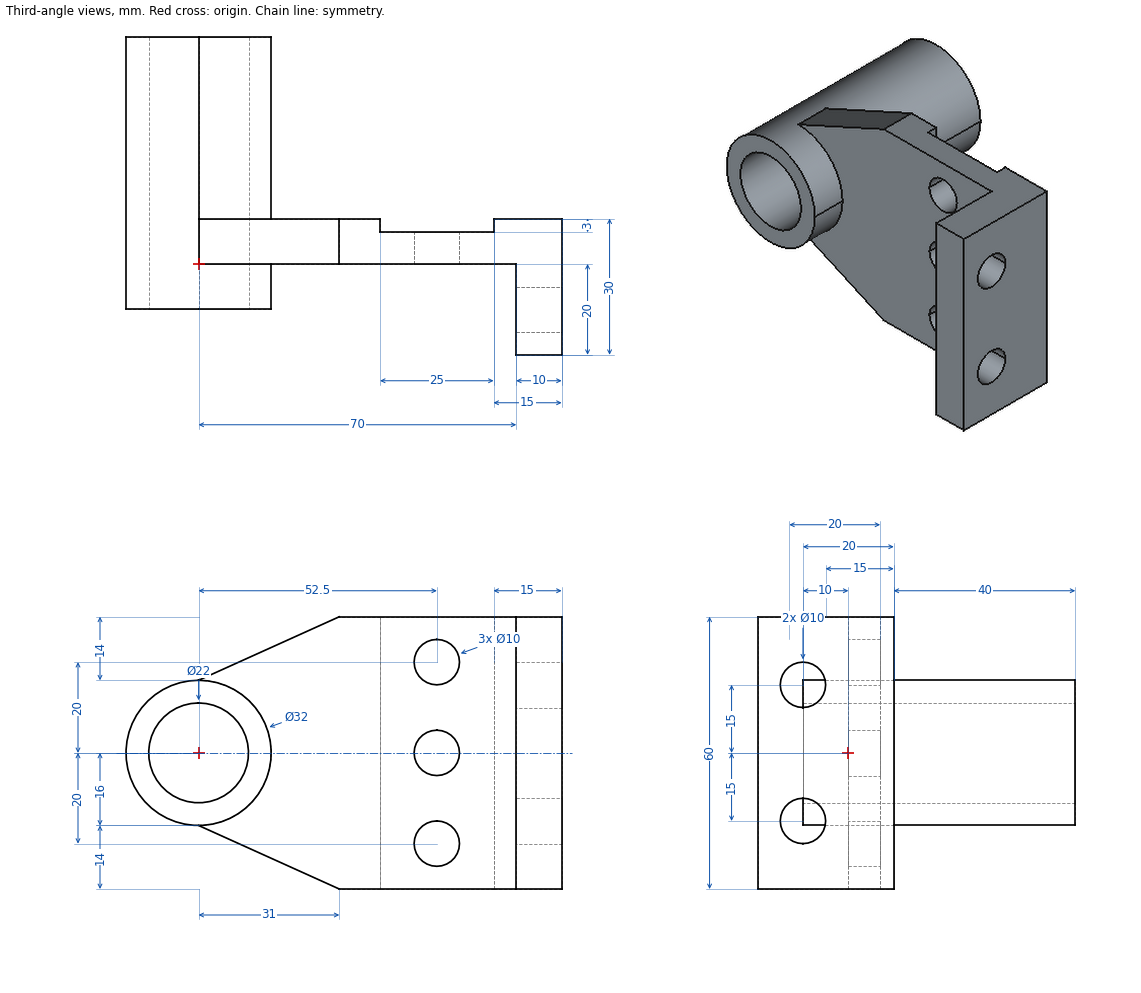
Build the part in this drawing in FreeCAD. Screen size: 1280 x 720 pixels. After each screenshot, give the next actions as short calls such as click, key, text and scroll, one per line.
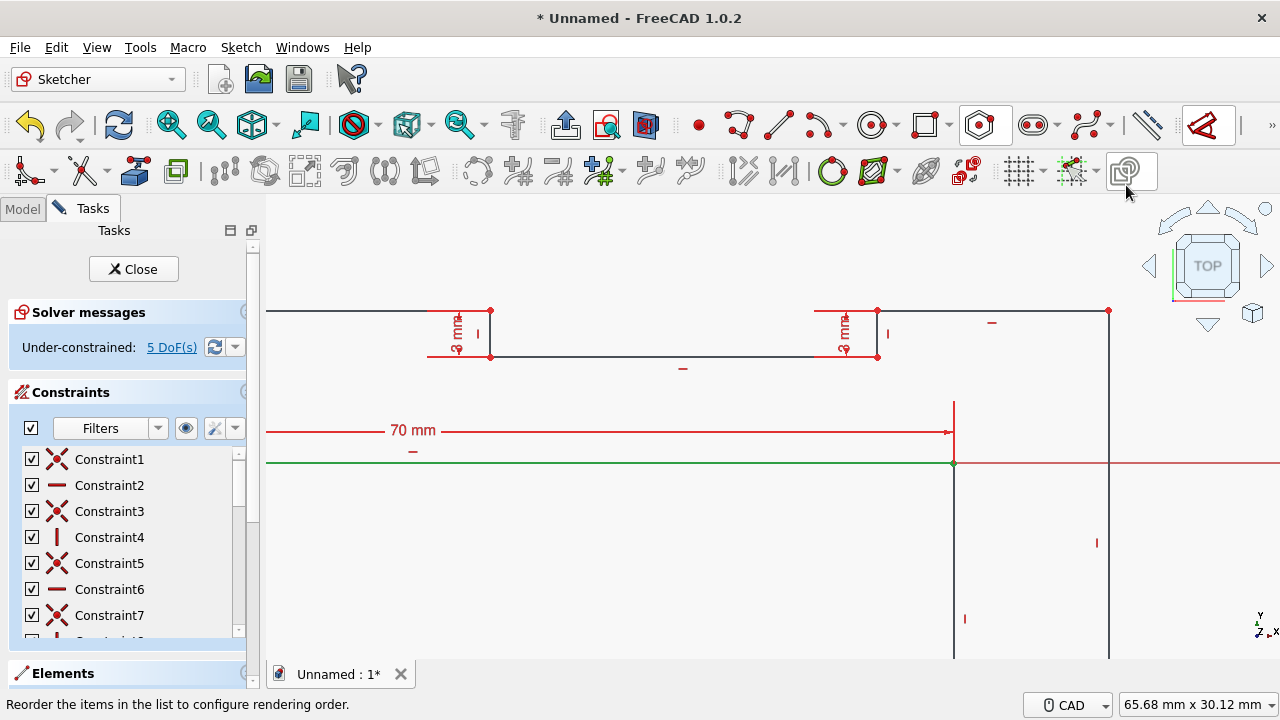
click(954, 556)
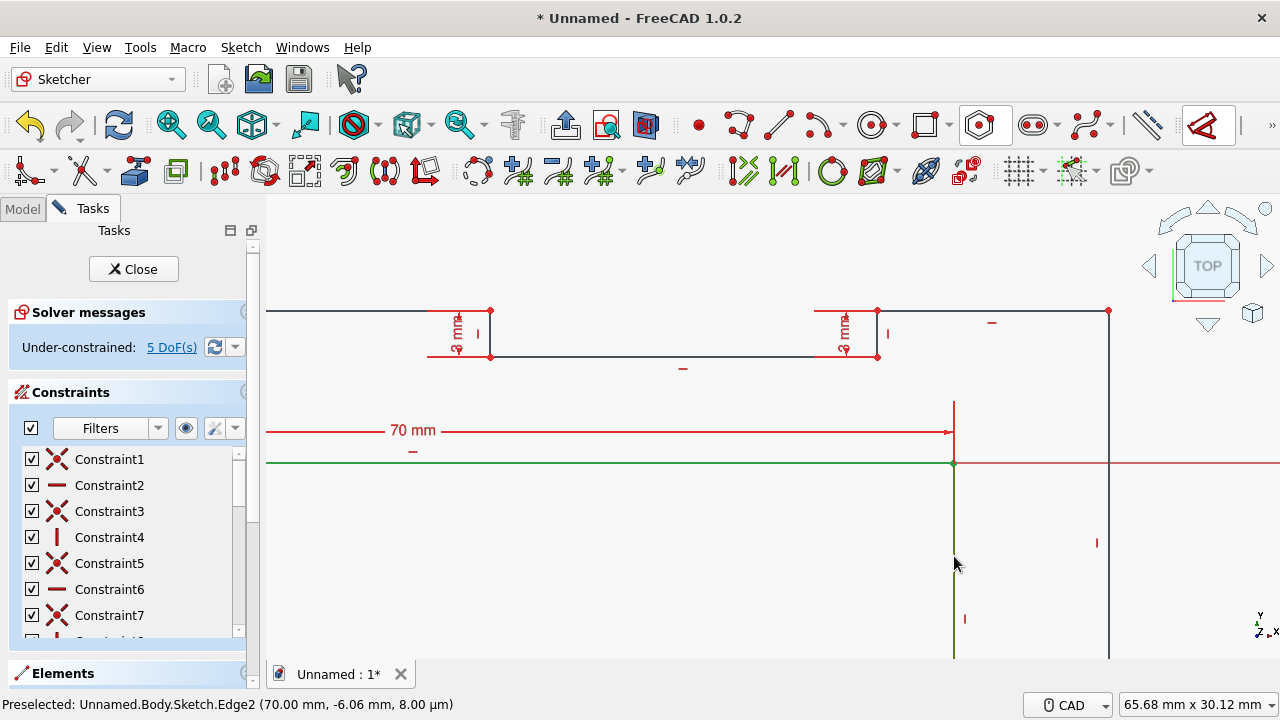
key(i)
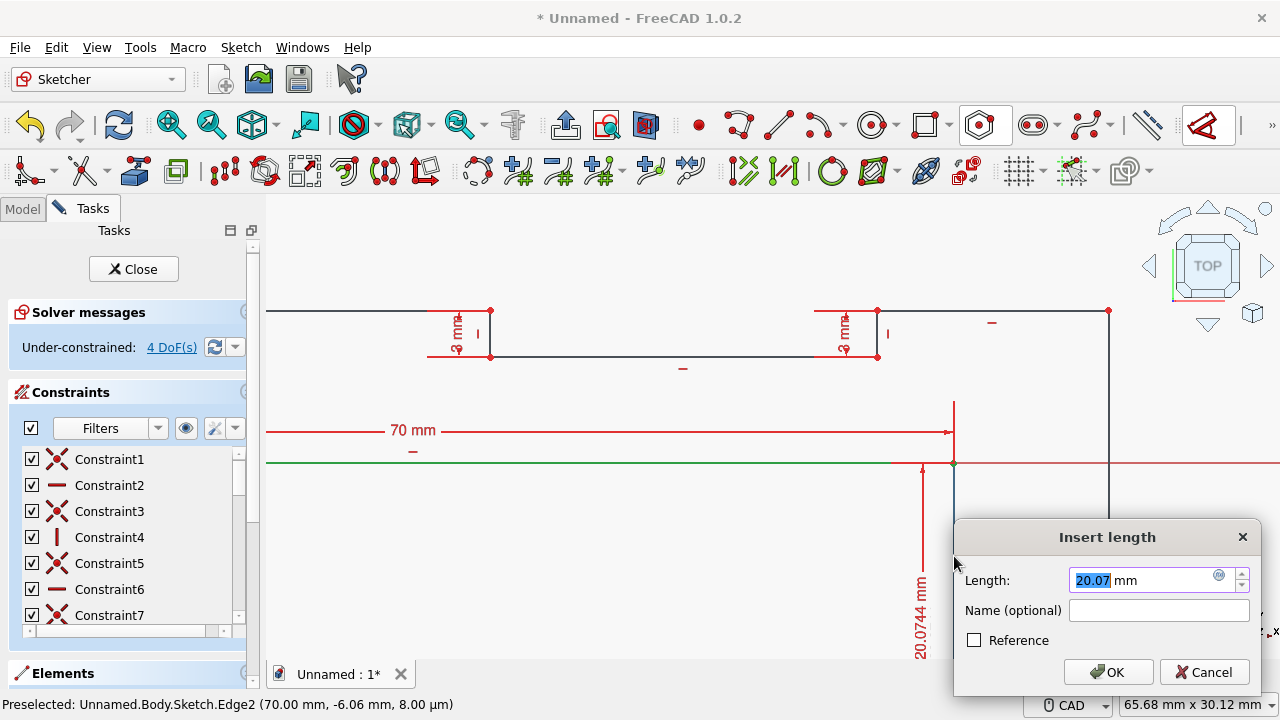
text(20)
key(Return)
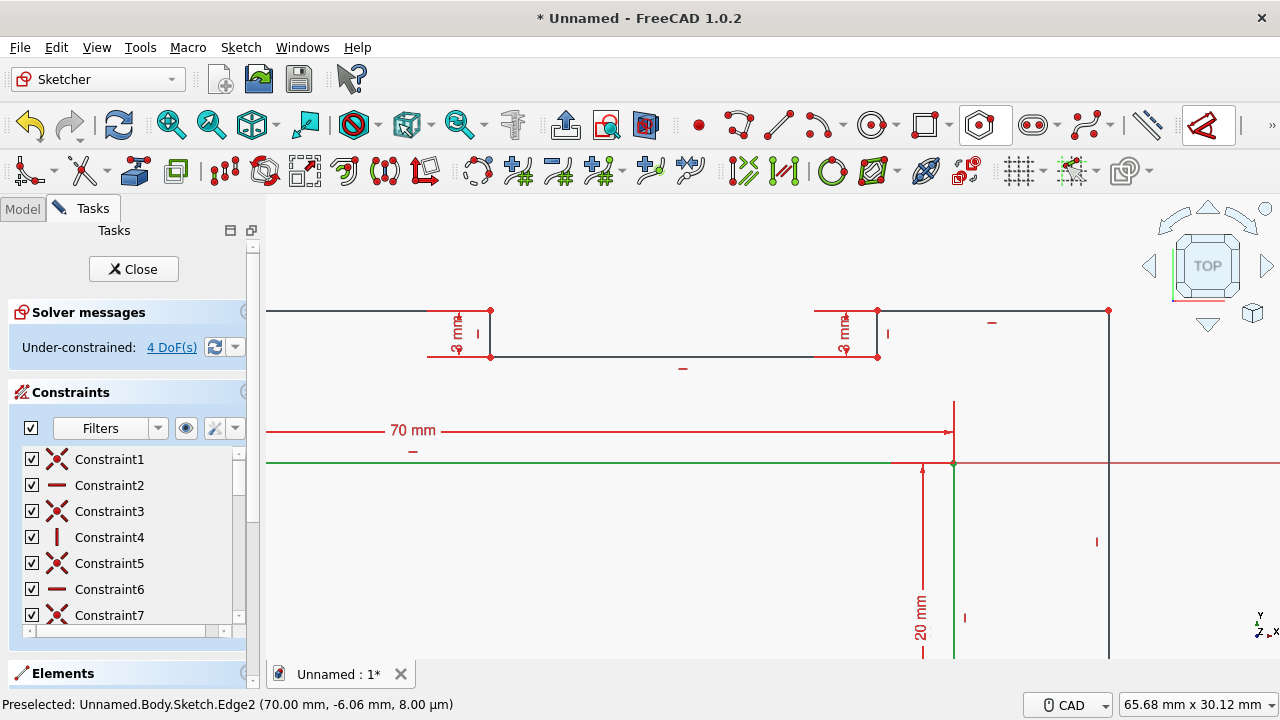
scroll(879, 333, down, 4)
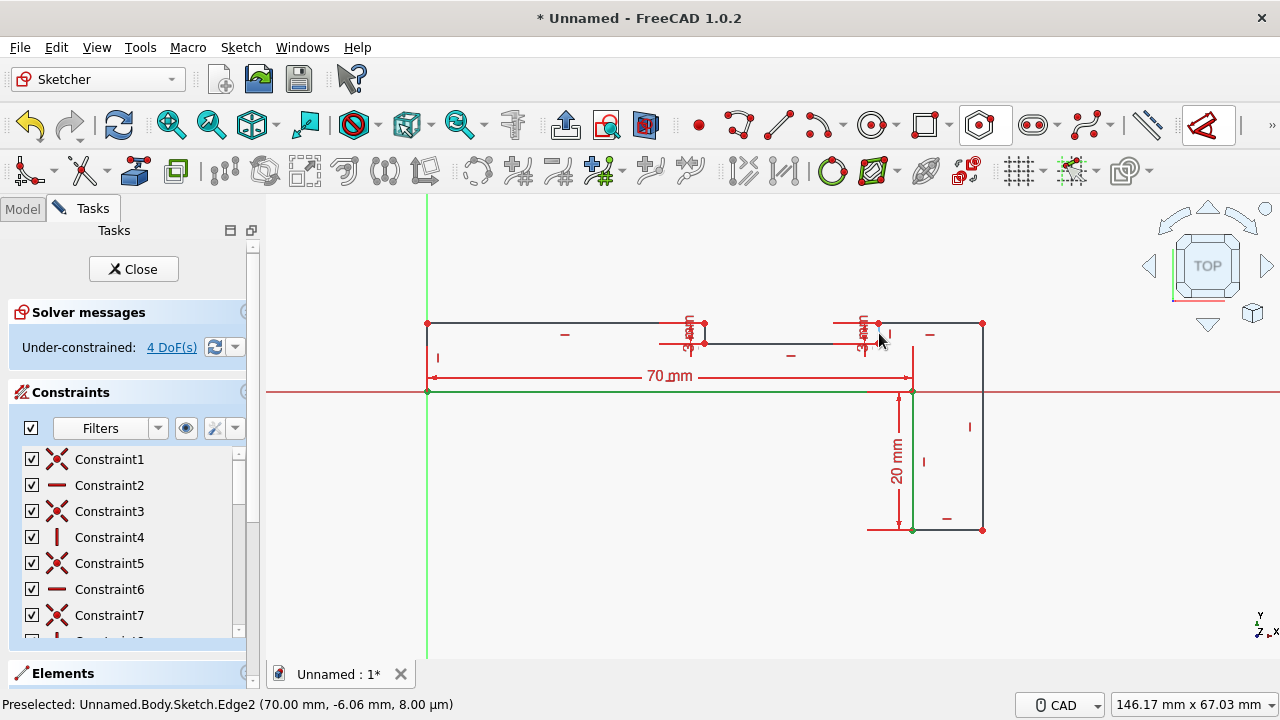
click(934, 530)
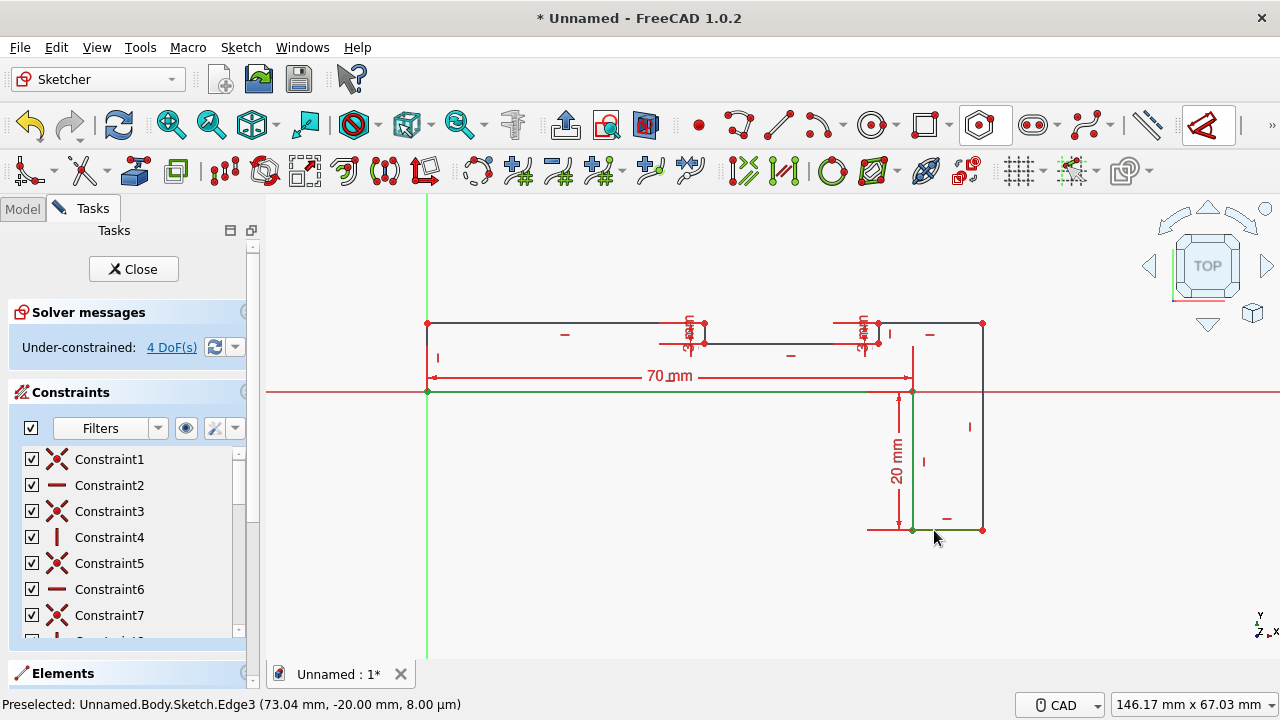
key(l)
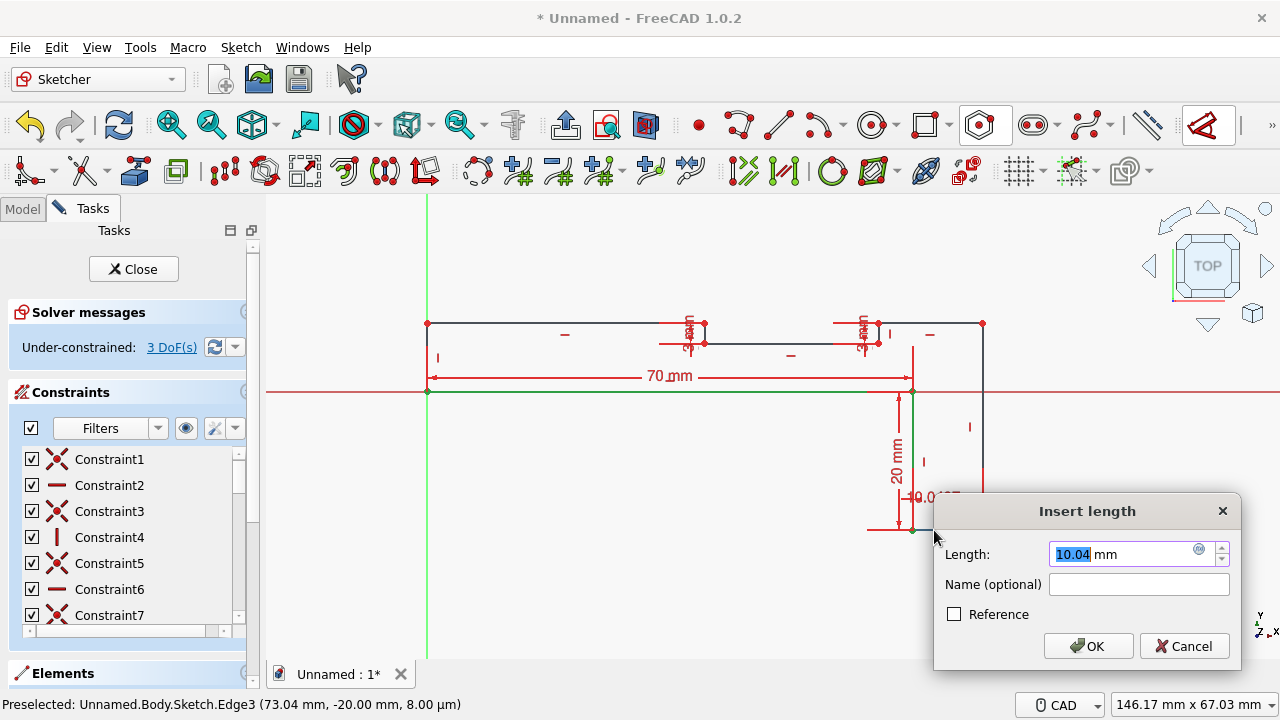
text(10)
key(Return)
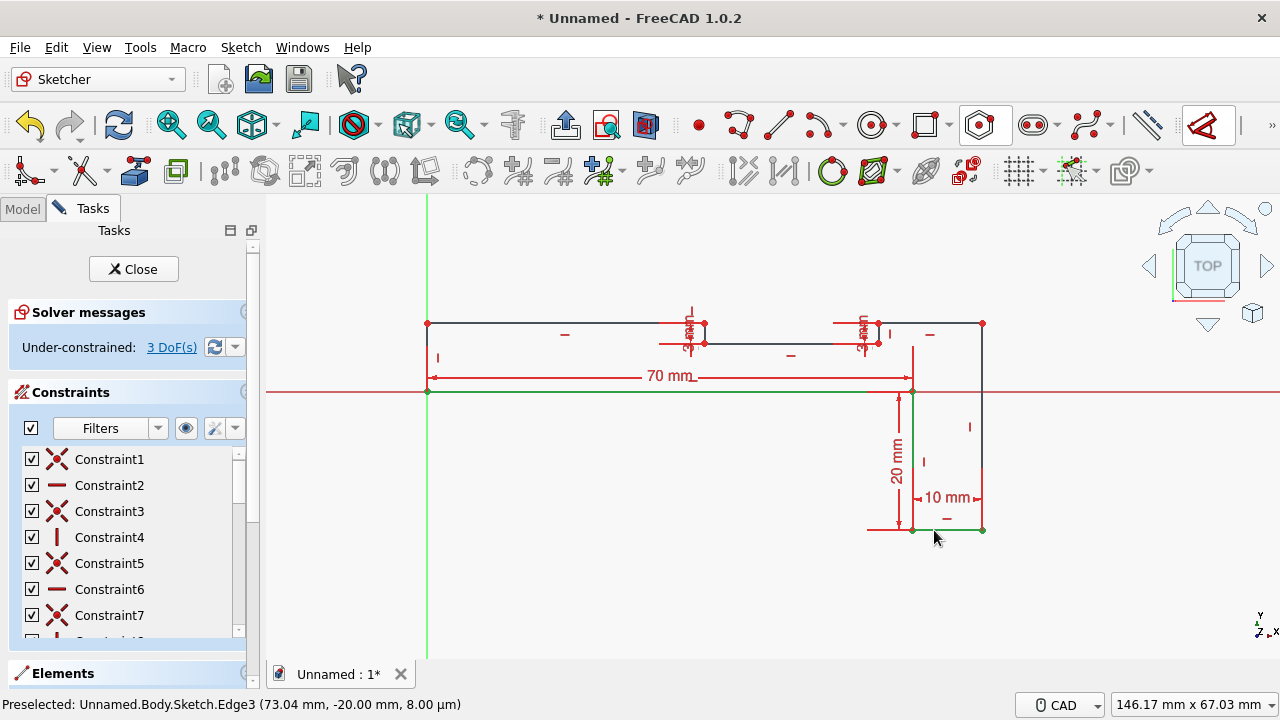
click(982, 468)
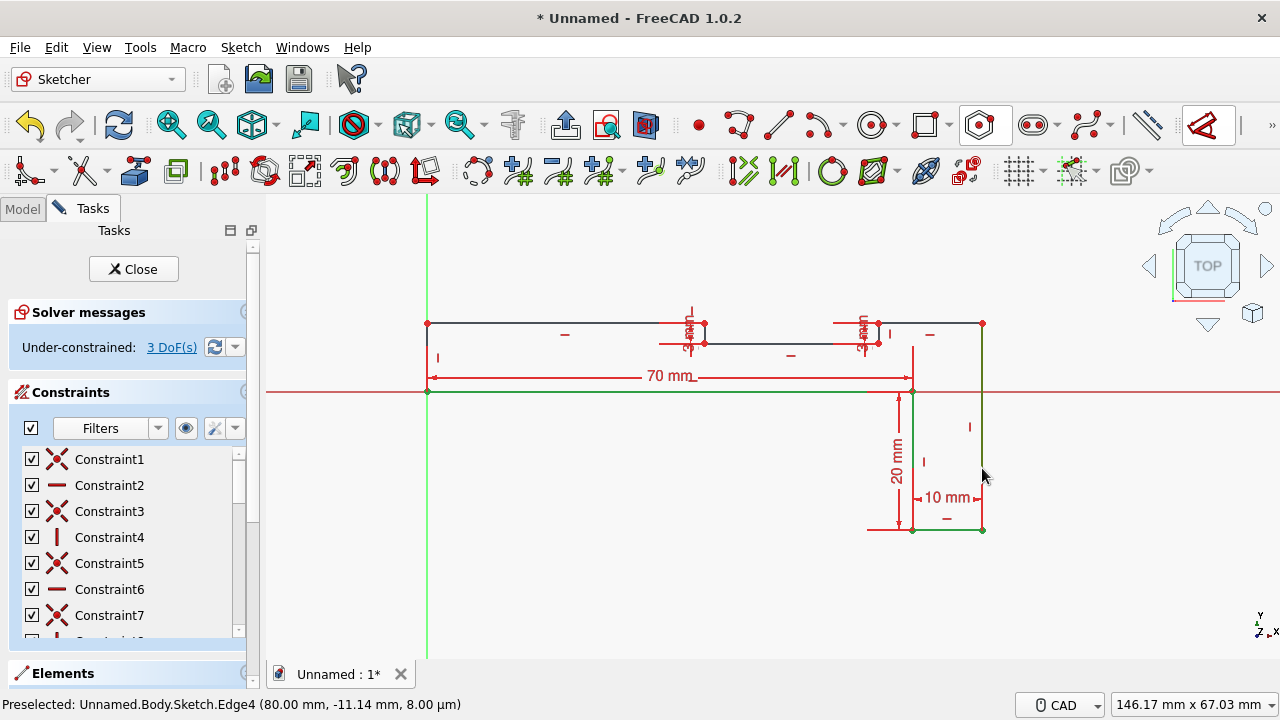
key(i)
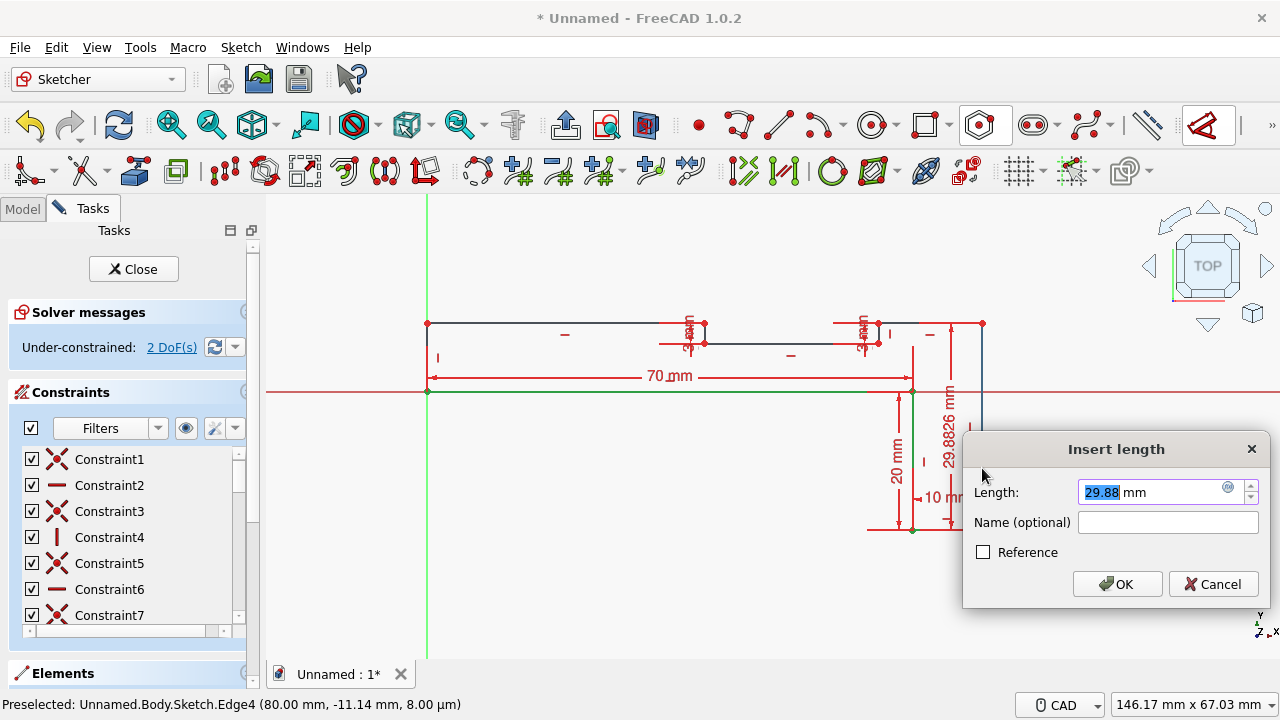
text(30)
key(Return)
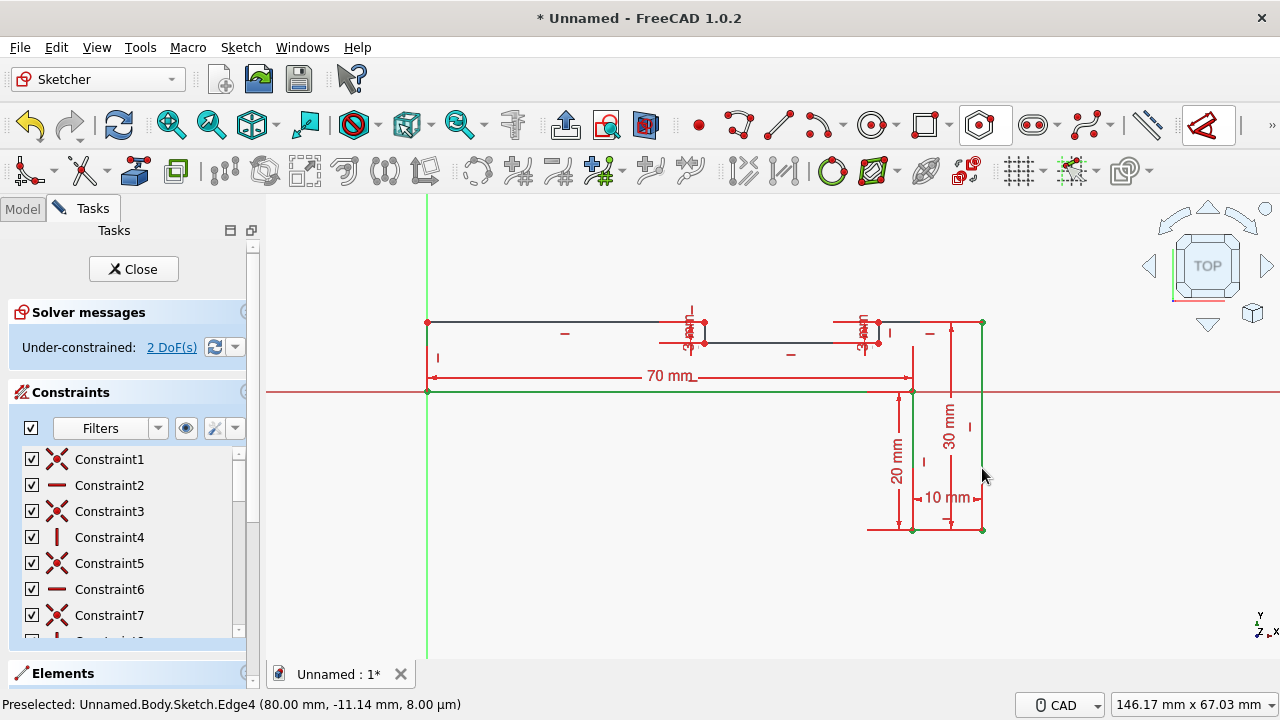
click(951, 322)